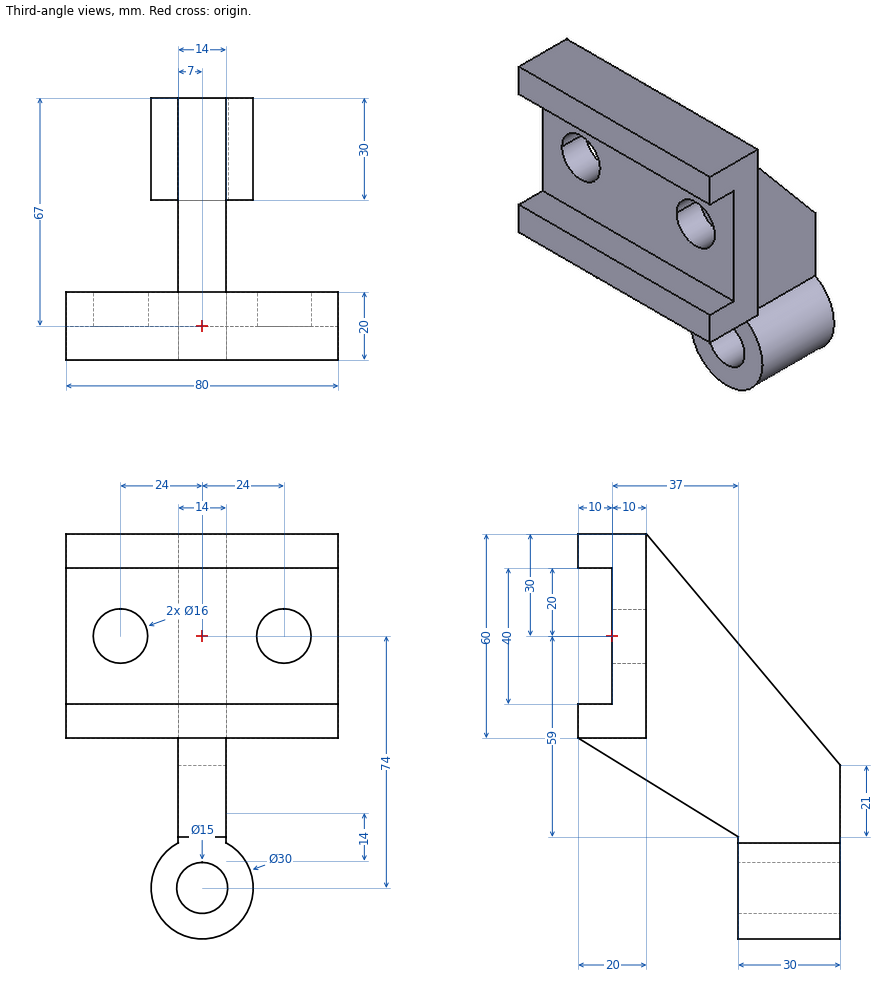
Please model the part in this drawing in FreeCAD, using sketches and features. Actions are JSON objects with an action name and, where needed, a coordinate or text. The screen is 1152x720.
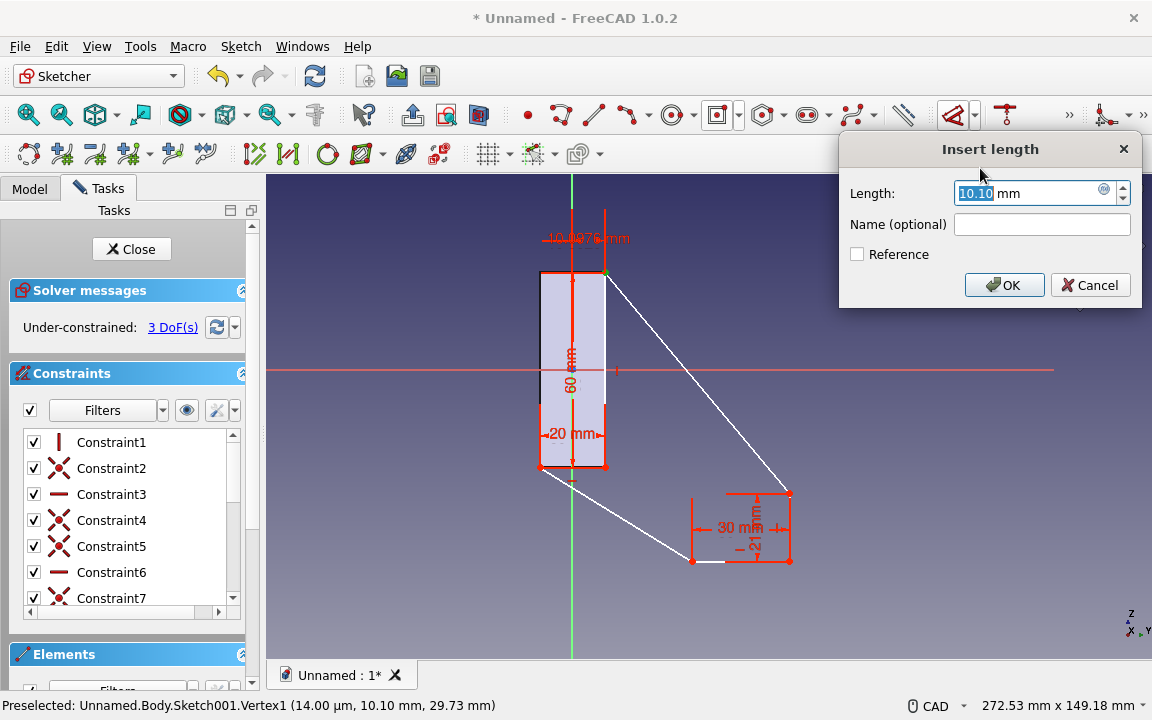
{"action": "type", "text": "10"}
{"action": "key", "text": "Return"}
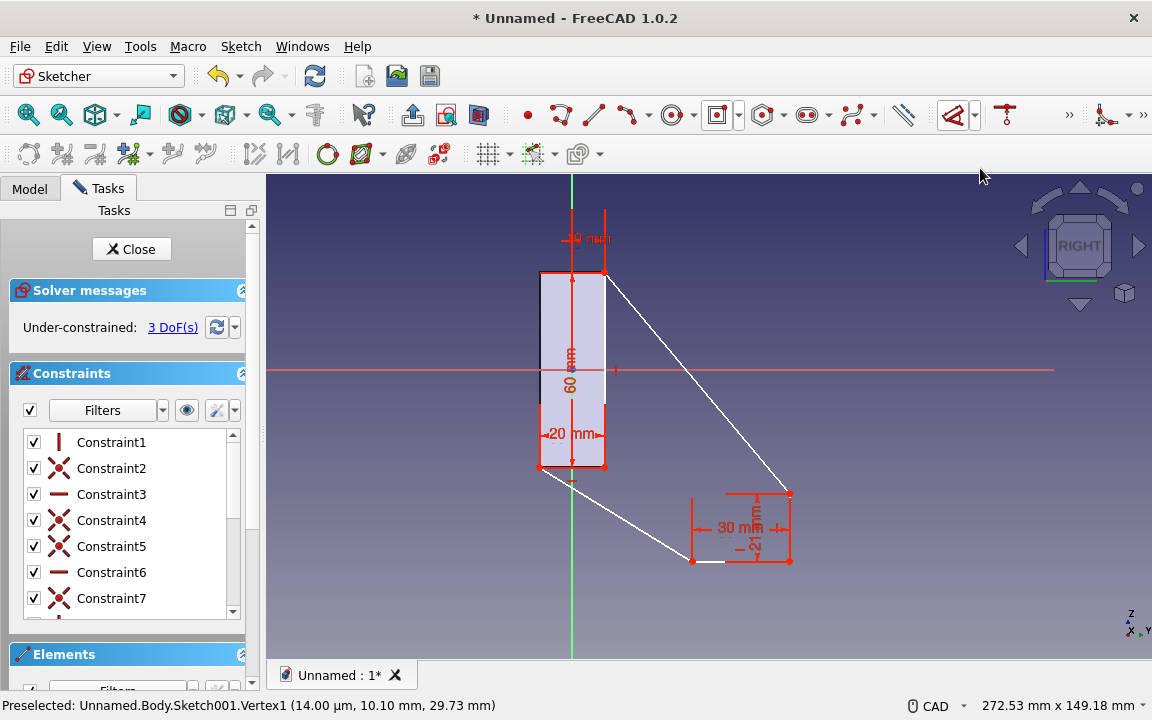
{"action": "left_click", "coordinate": [605, 273]}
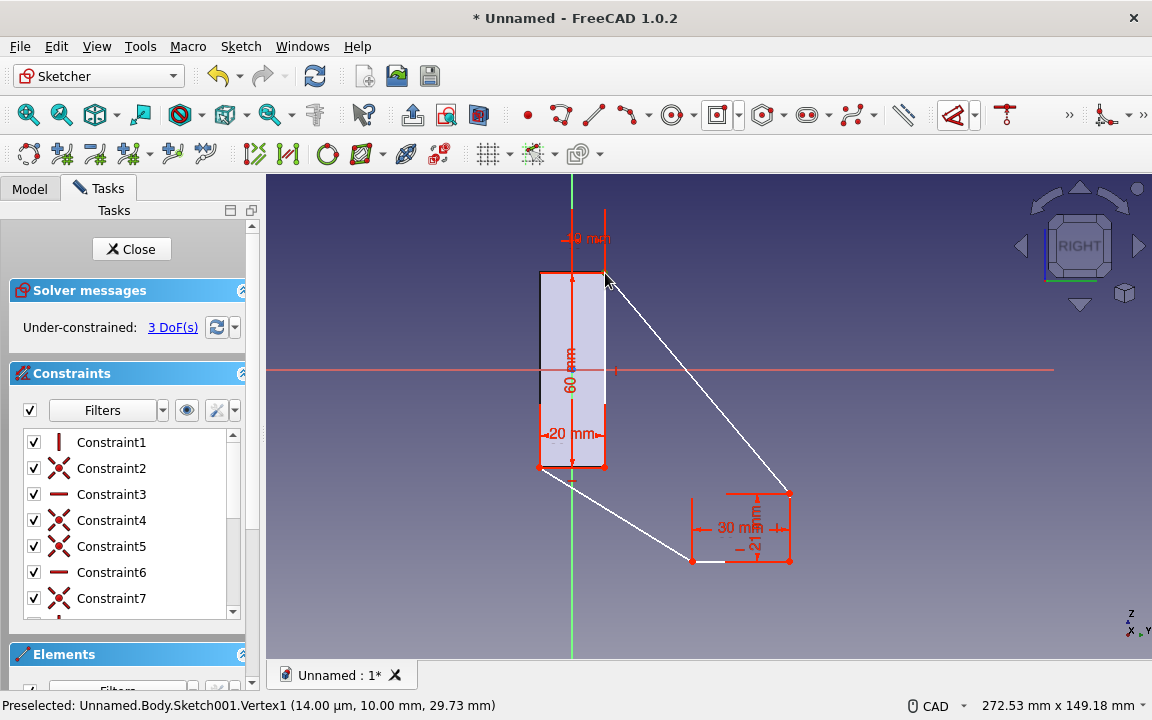
{"action": "left_click", "coordinate": [974, 116]}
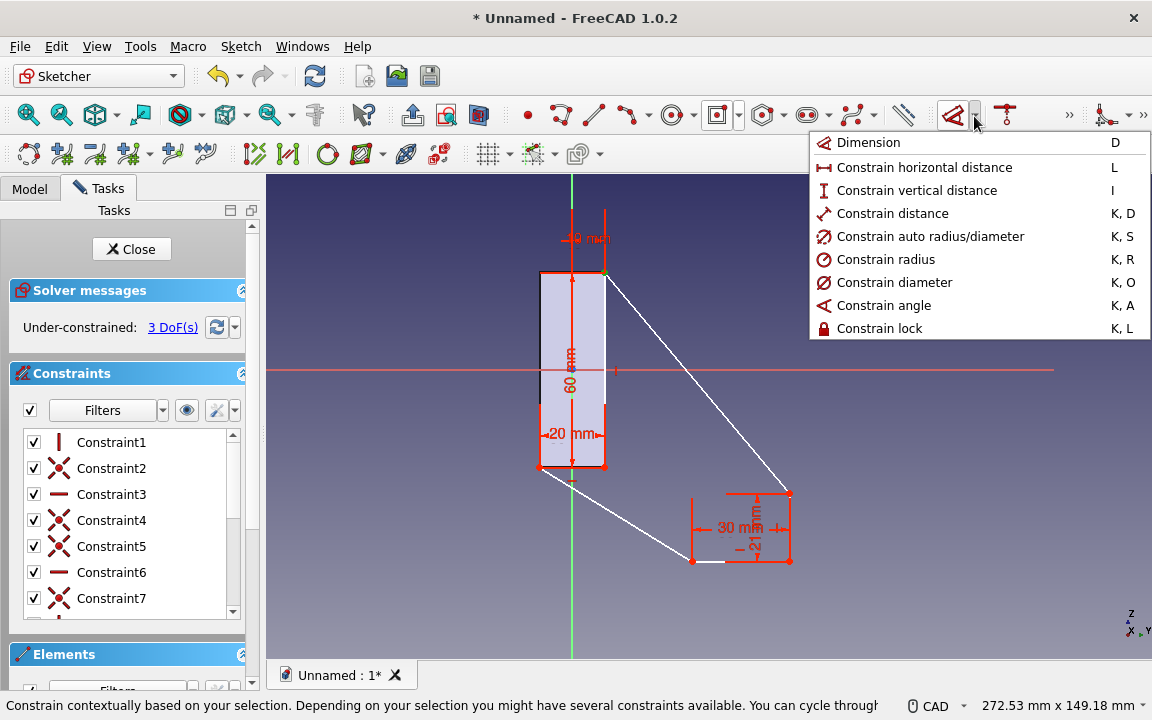
{"action": "left_click", "coordinate": [980, 190]}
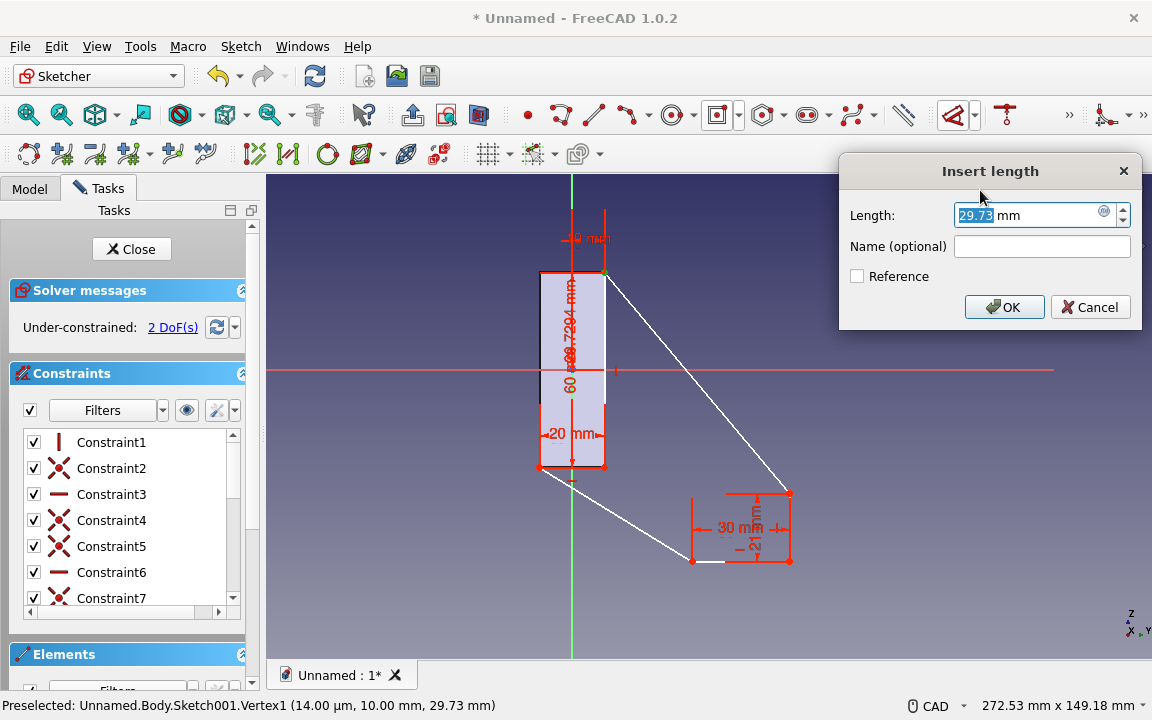
{"action": "type", "text": "30"}
{"action": "key", "text": "Return"}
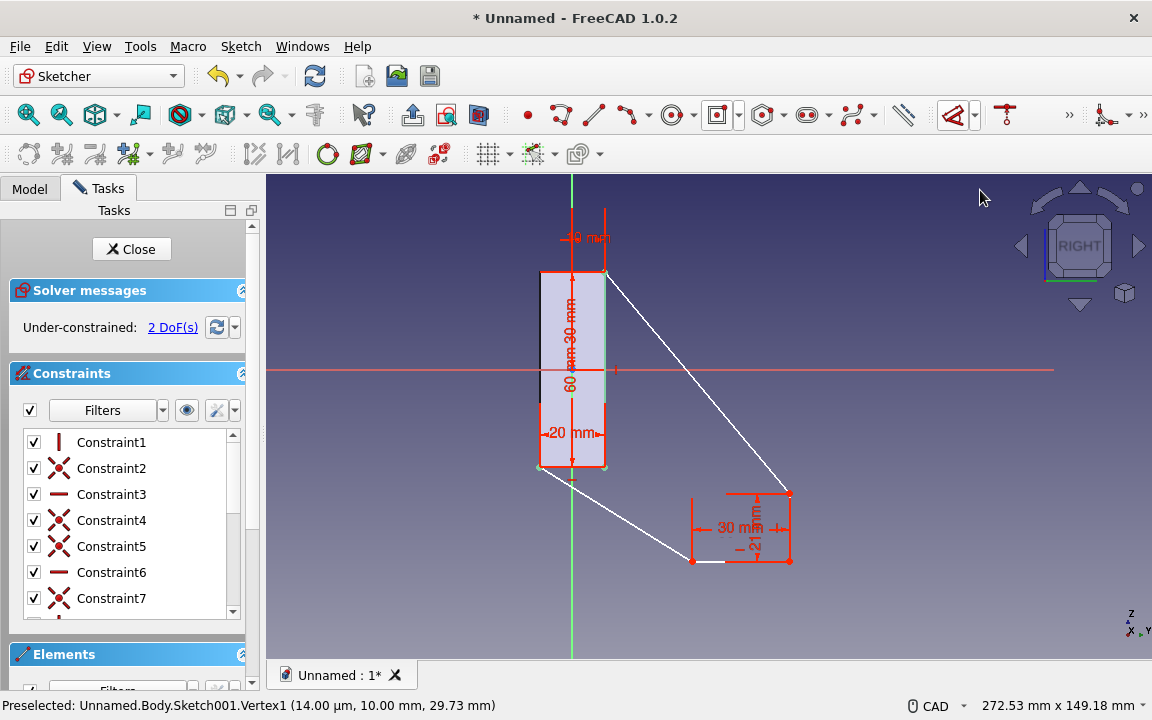
{"action": "left_click", "coordinate": [692, 562]}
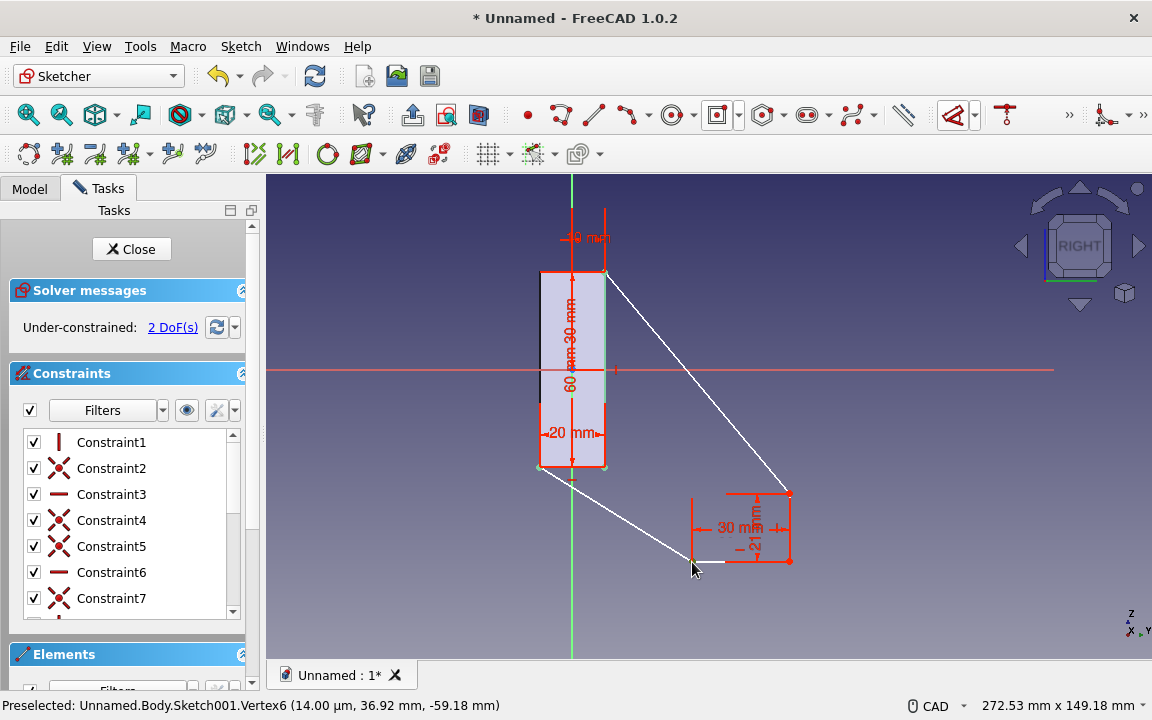
{"action": "left_click", "coordinate": [974, 116]}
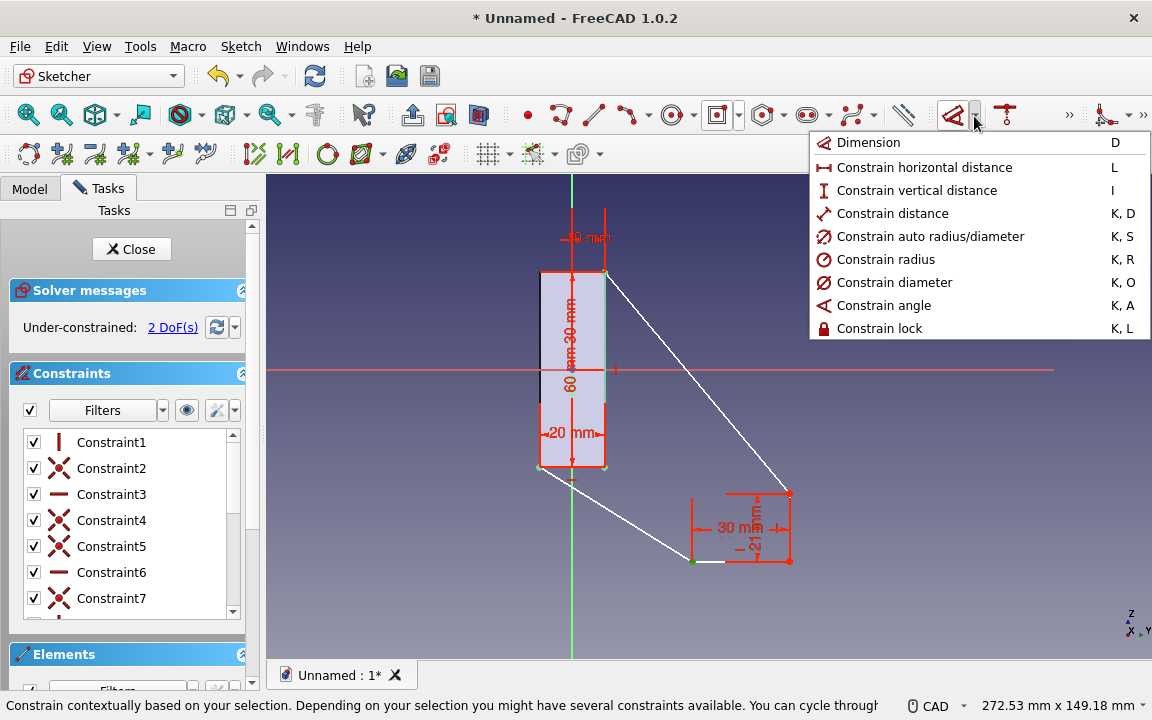
{"action": "left_click", "coordinate": [980, 168]}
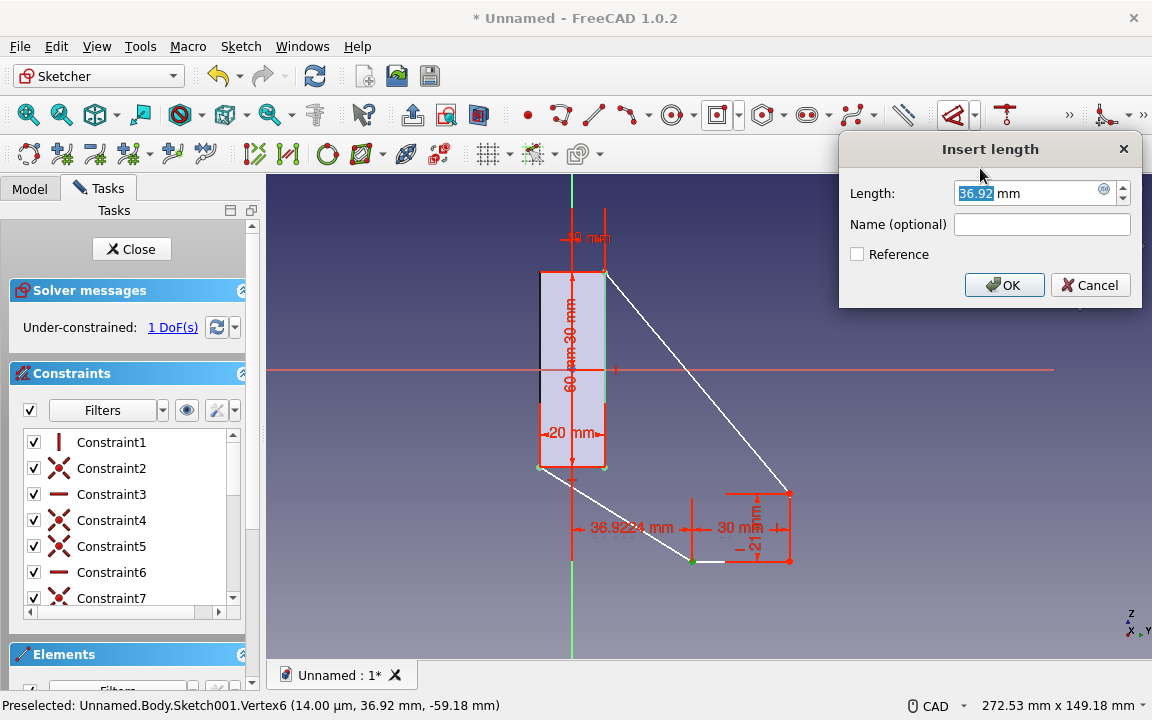
{"action": "type", "text": "37"}
{"action": "key", "text": "Return"}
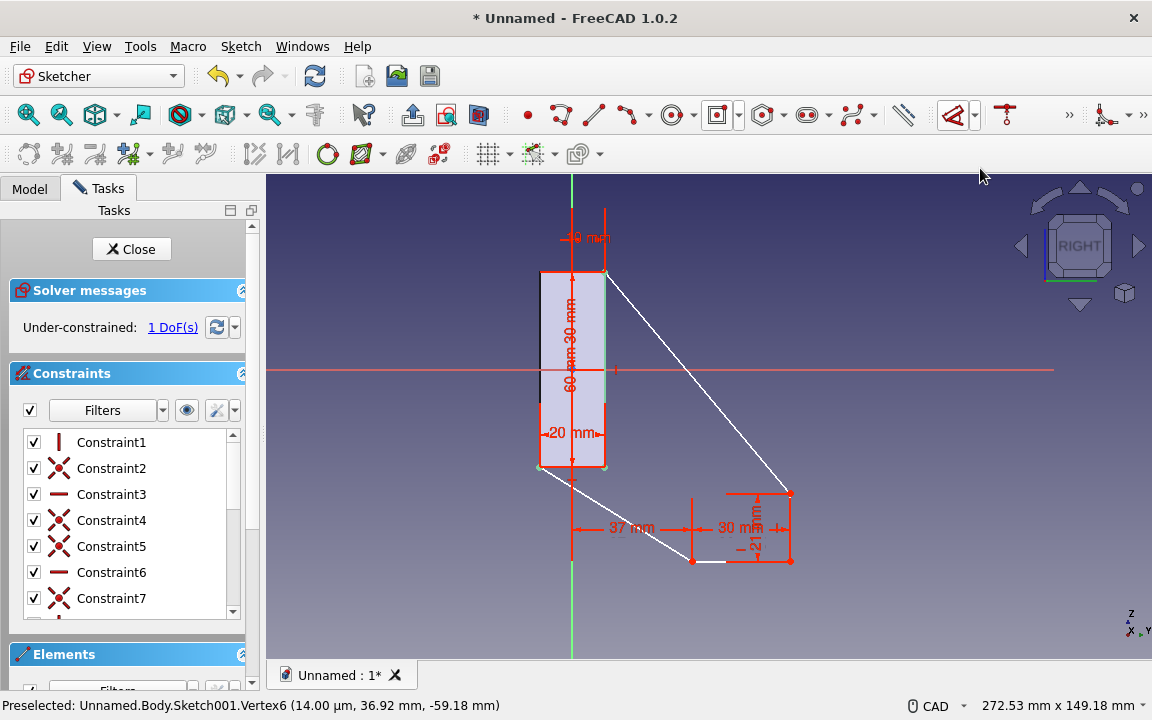
{"action": "left_click", "coordinate": [692, 562]}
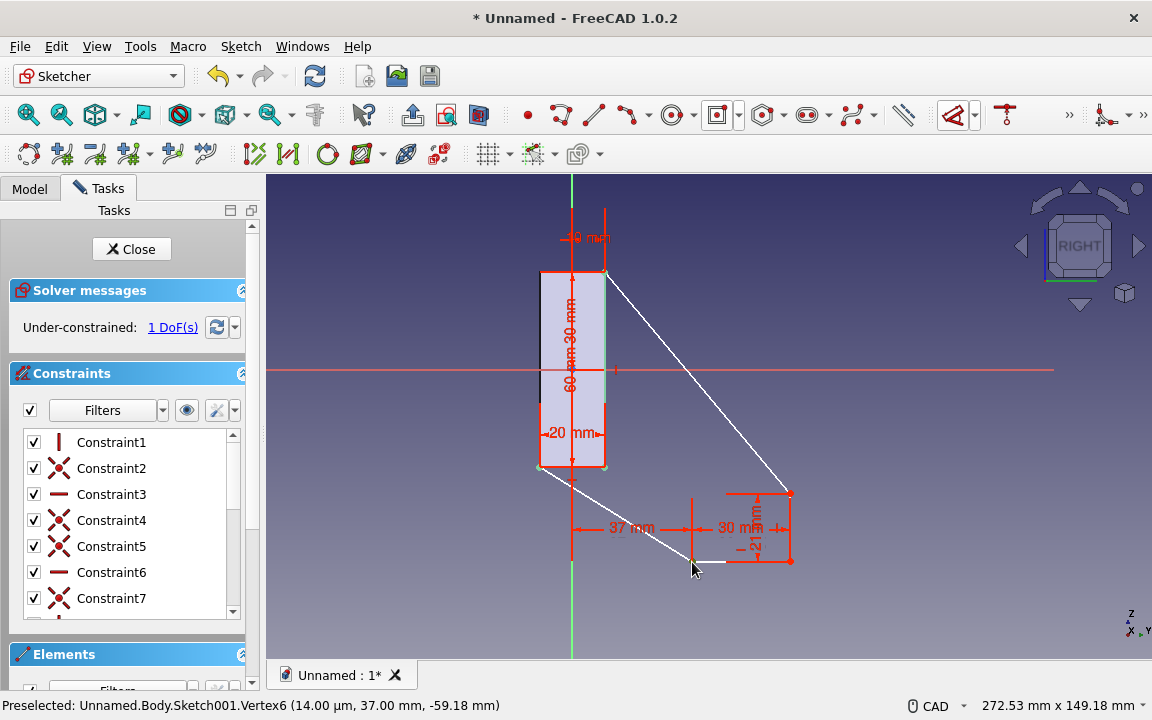
{"action": "key", "text": "i"}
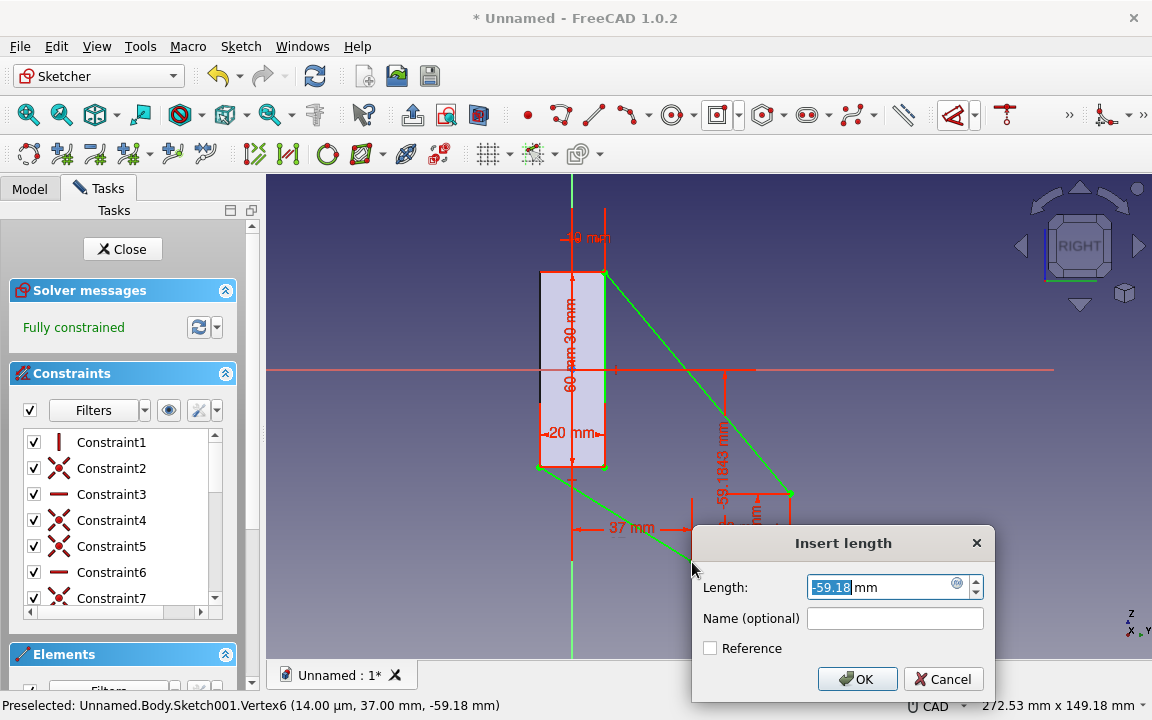
{"action": "type", "text": "-59"}
{"action": "key", "text": "Return"}